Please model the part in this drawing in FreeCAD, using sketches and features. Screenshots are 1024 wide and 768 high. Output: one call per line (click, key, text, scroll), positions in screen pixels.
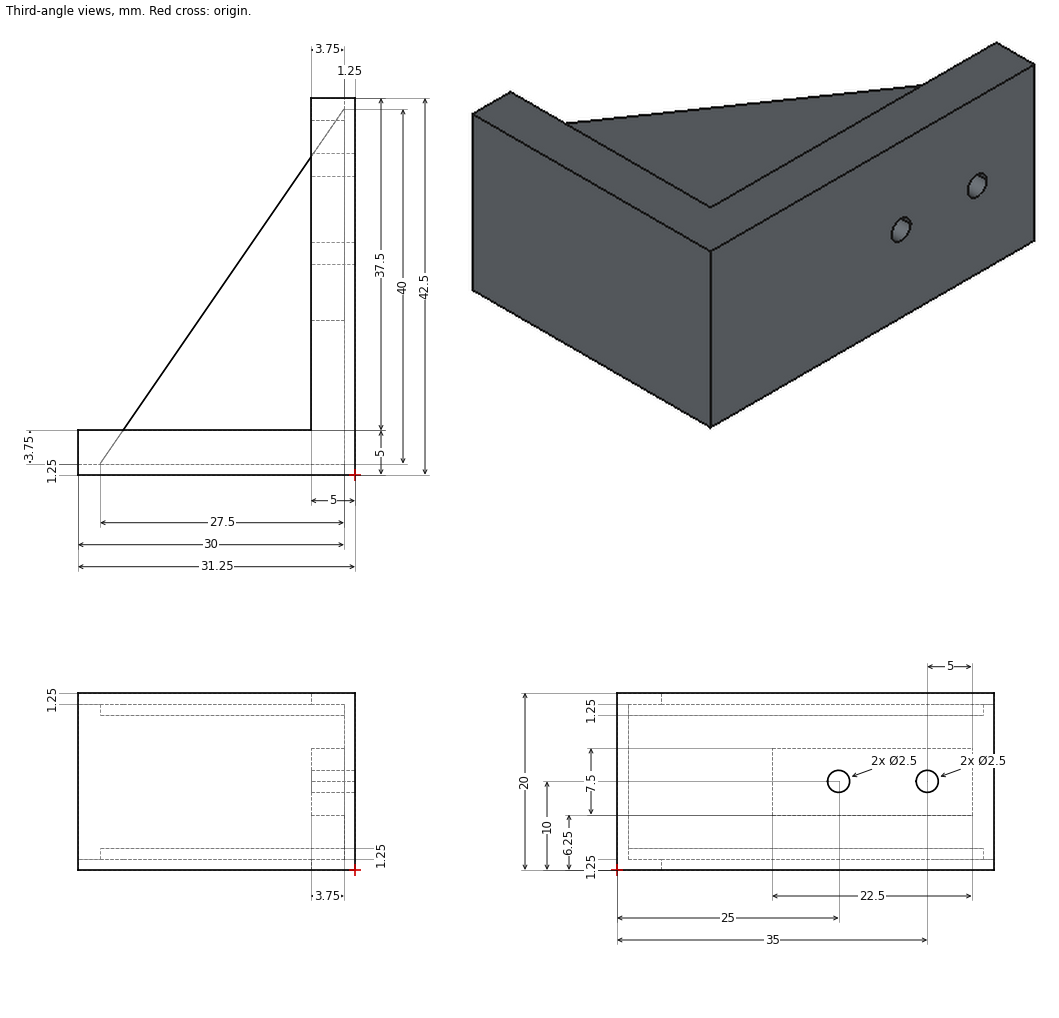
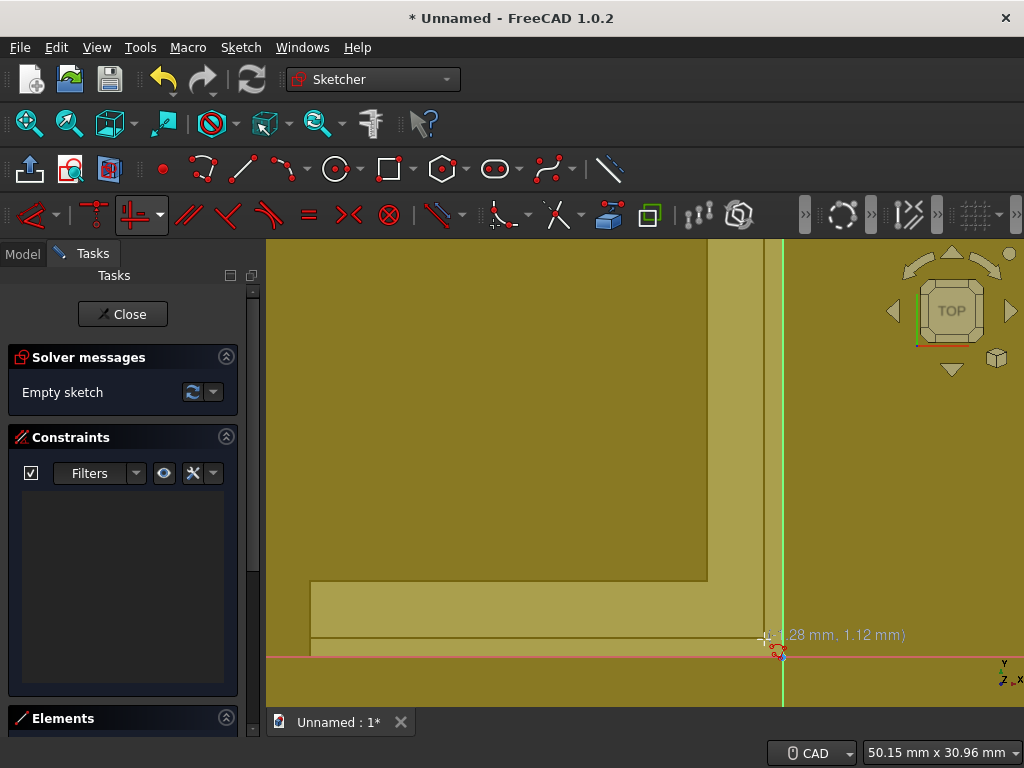
click(764, 638)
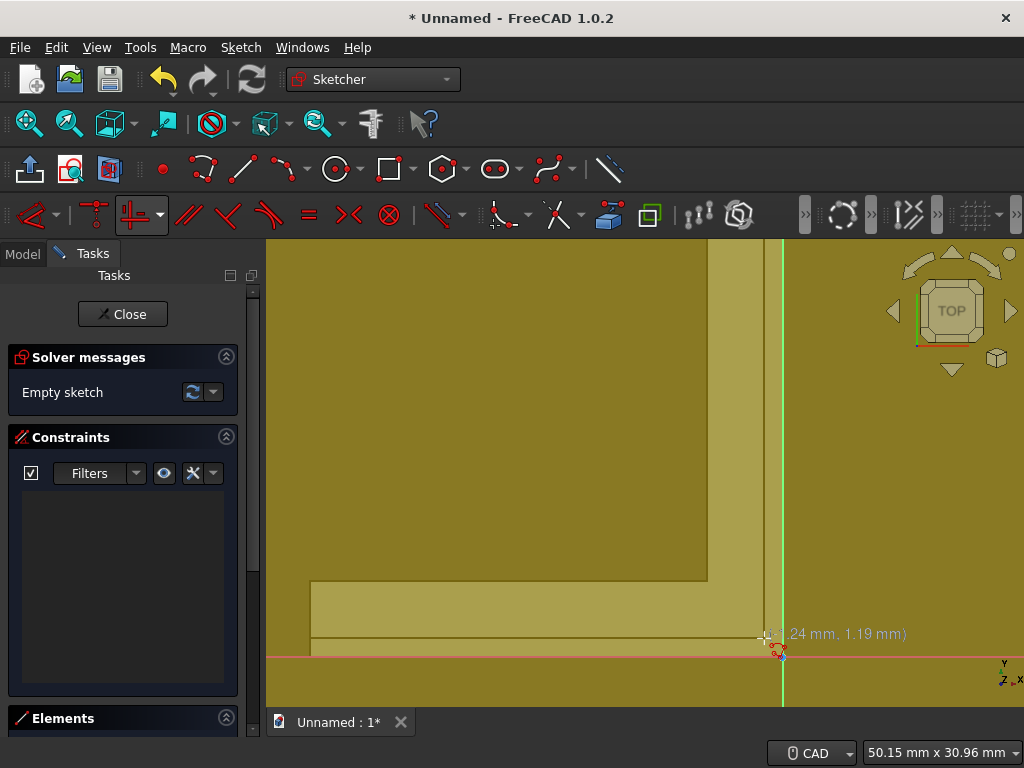
scroll(585, 577, down, 4)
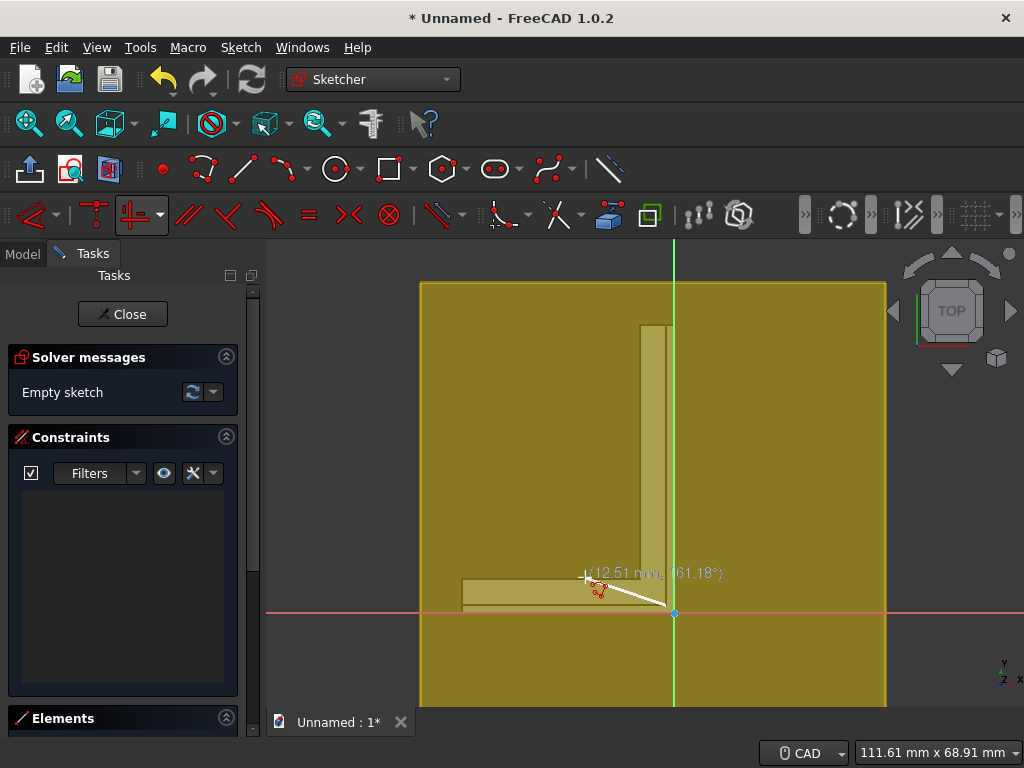
scroll(666, 333, up, 4)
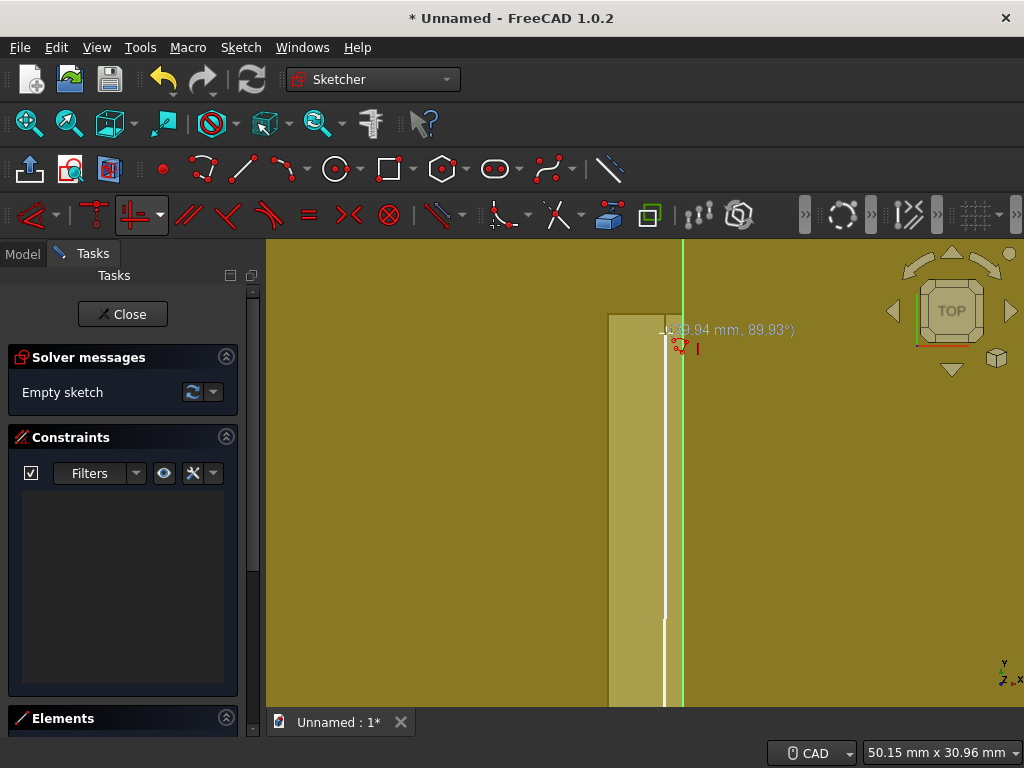
click(665, 333)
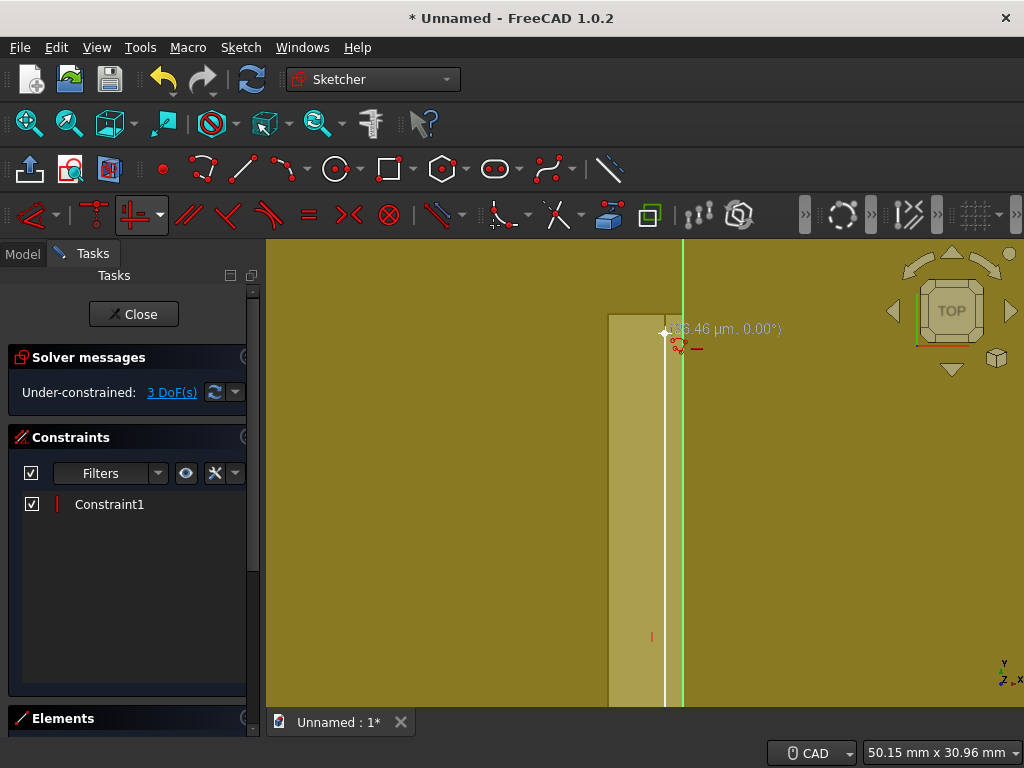
scroll(667, 333, down, 4)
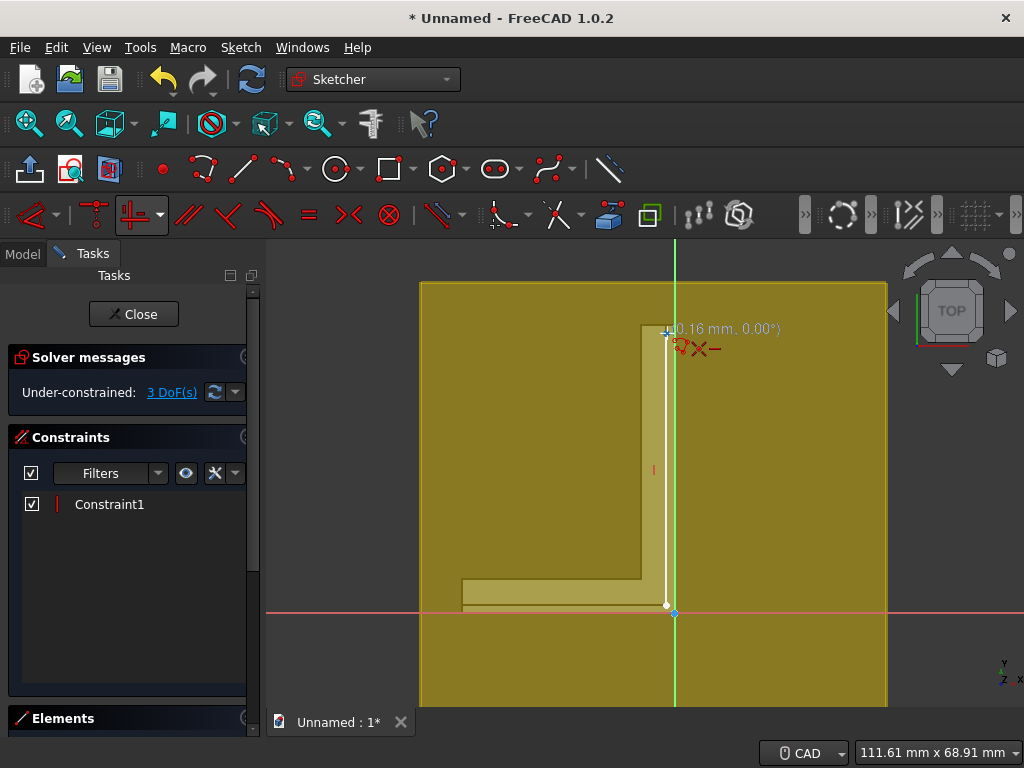
scroll(479, 605, up, 4)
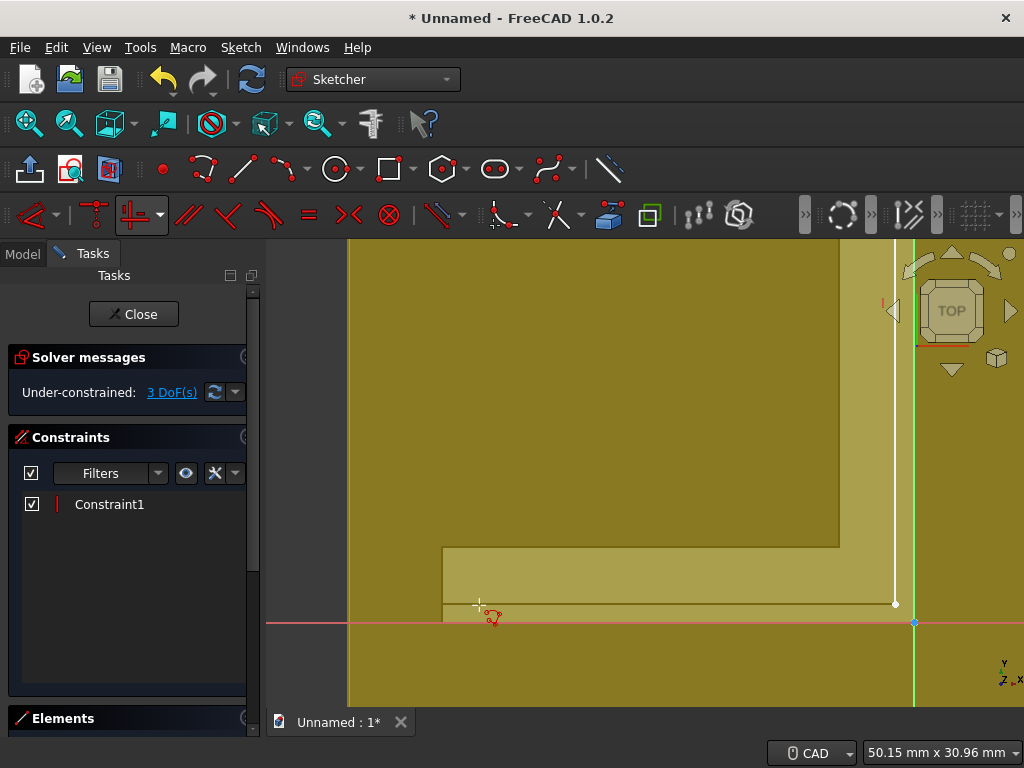
click(480, 604)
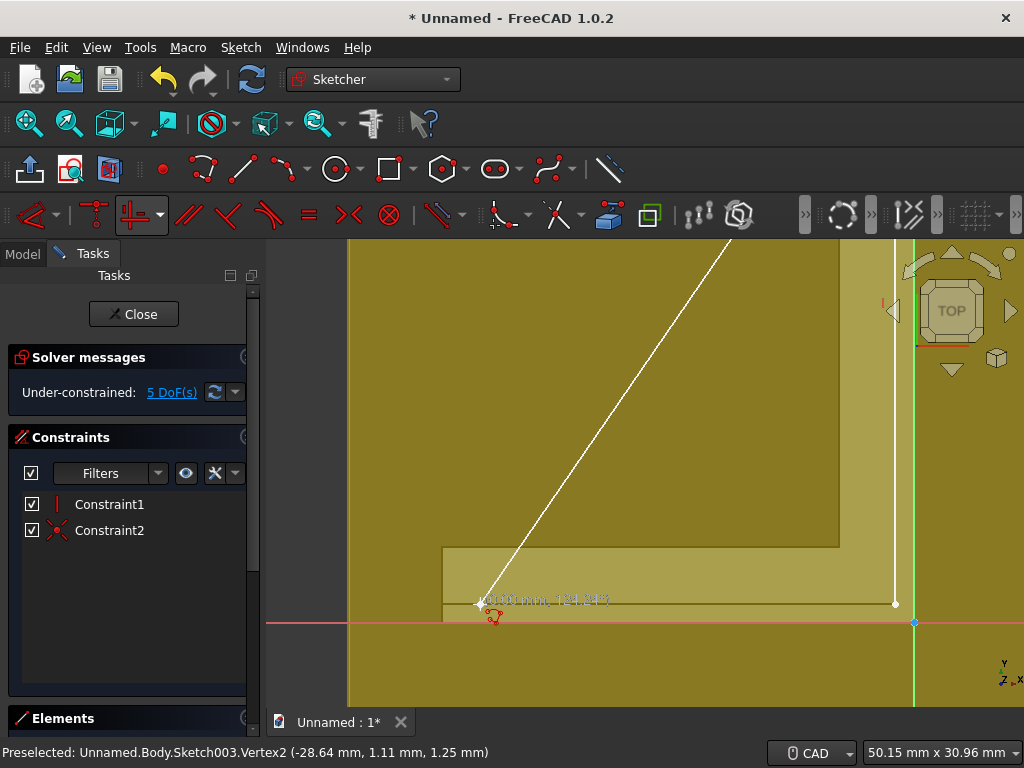
scroll(478, 605, down, 4)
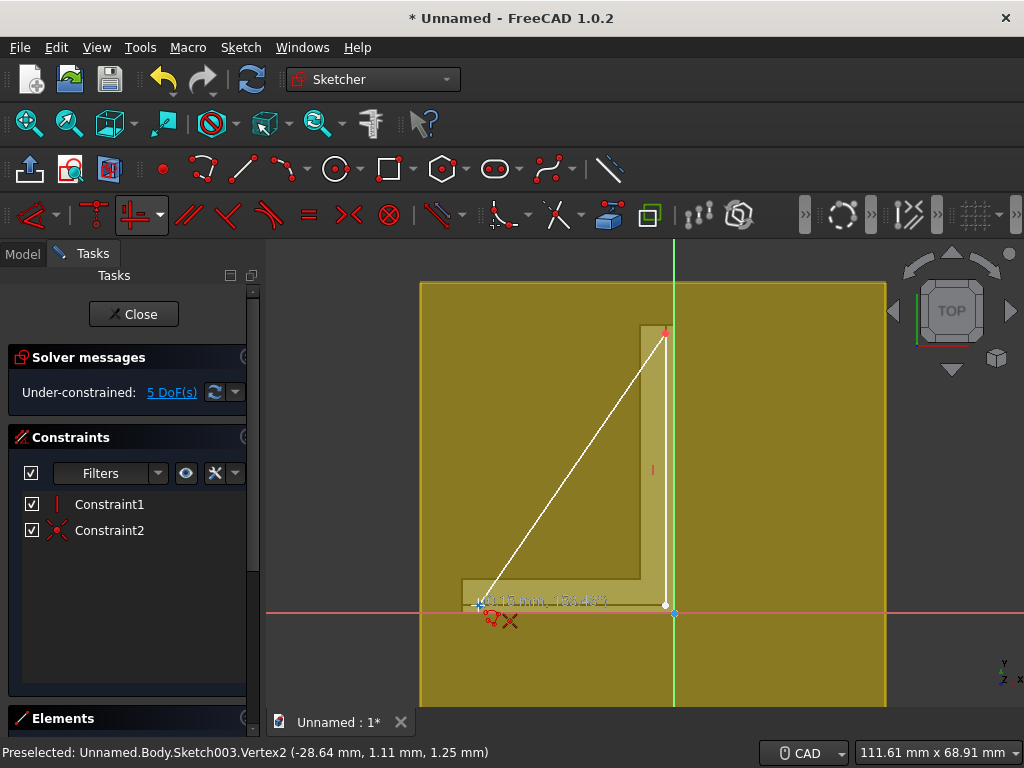
scroll(666, 605, up, 4)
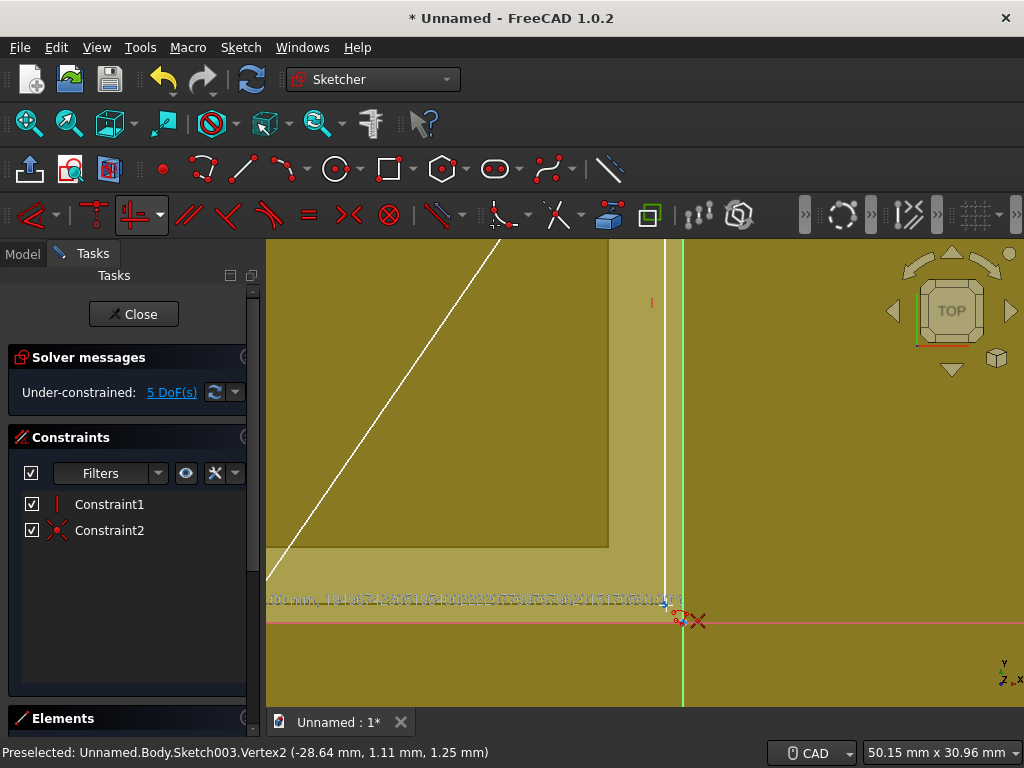
click(665, 605)
key(Escape)
key(Escape)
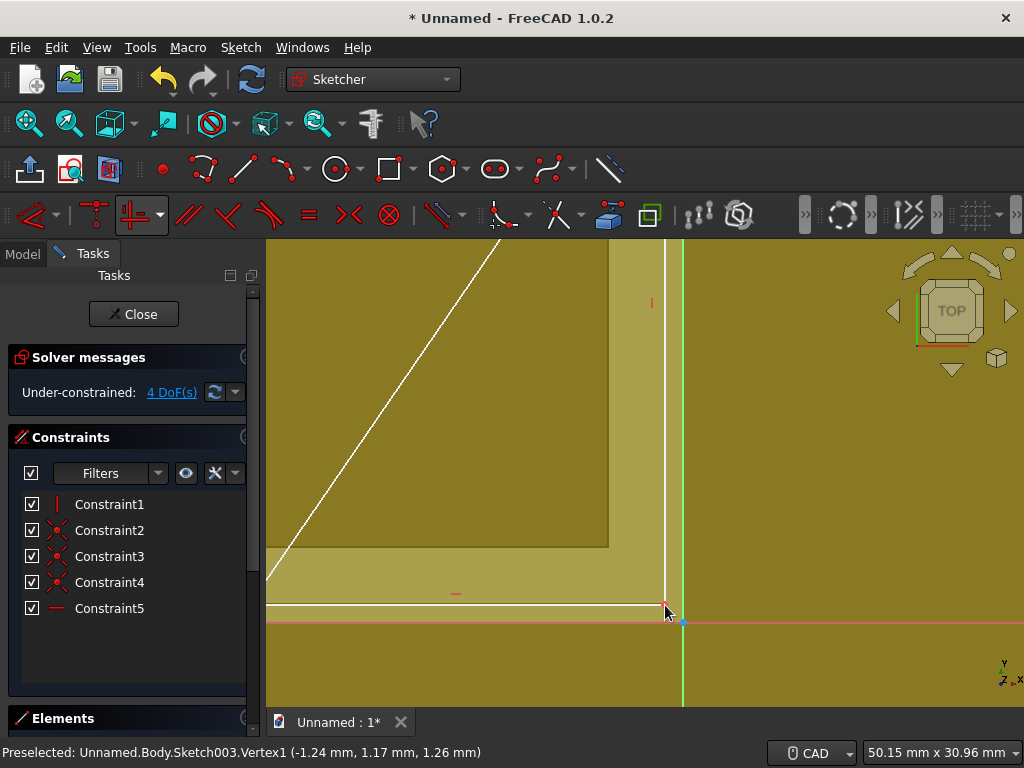
click(32, 216)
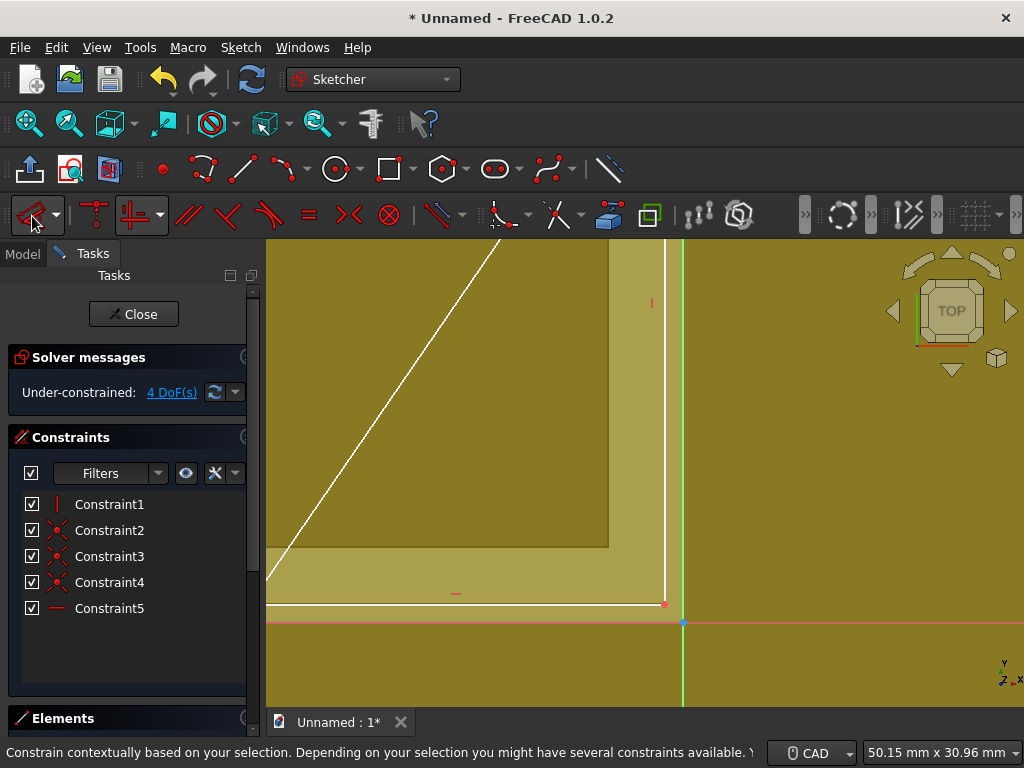
click(665, 423)
click(699, 436)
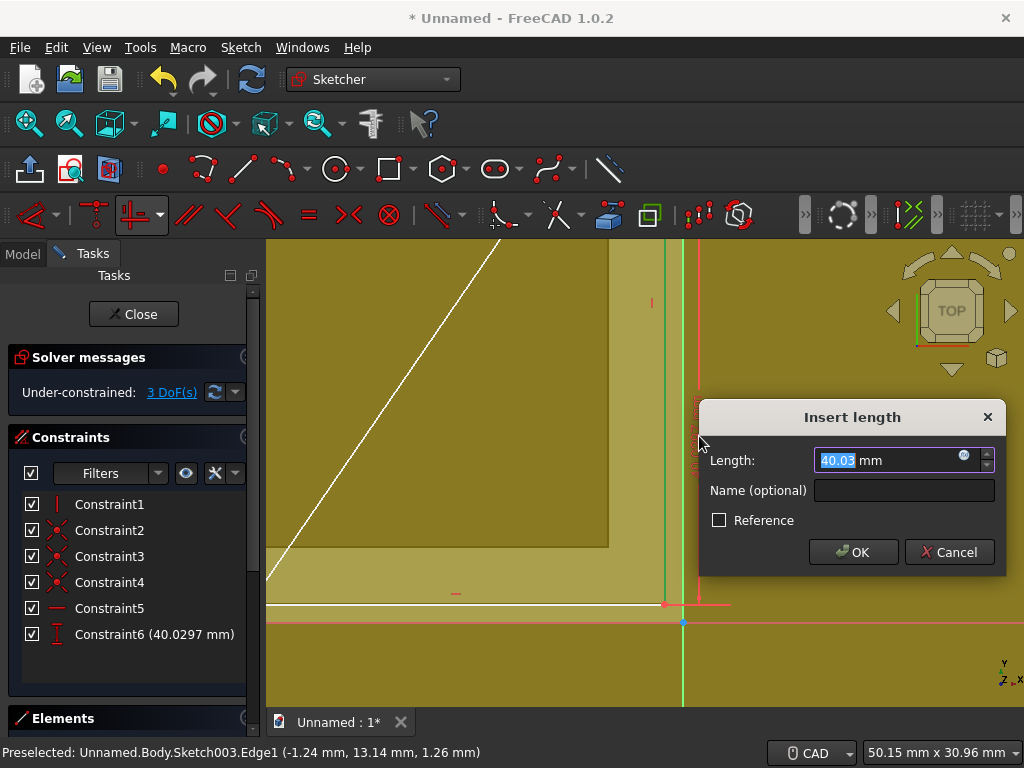
text(40)
key(Return)